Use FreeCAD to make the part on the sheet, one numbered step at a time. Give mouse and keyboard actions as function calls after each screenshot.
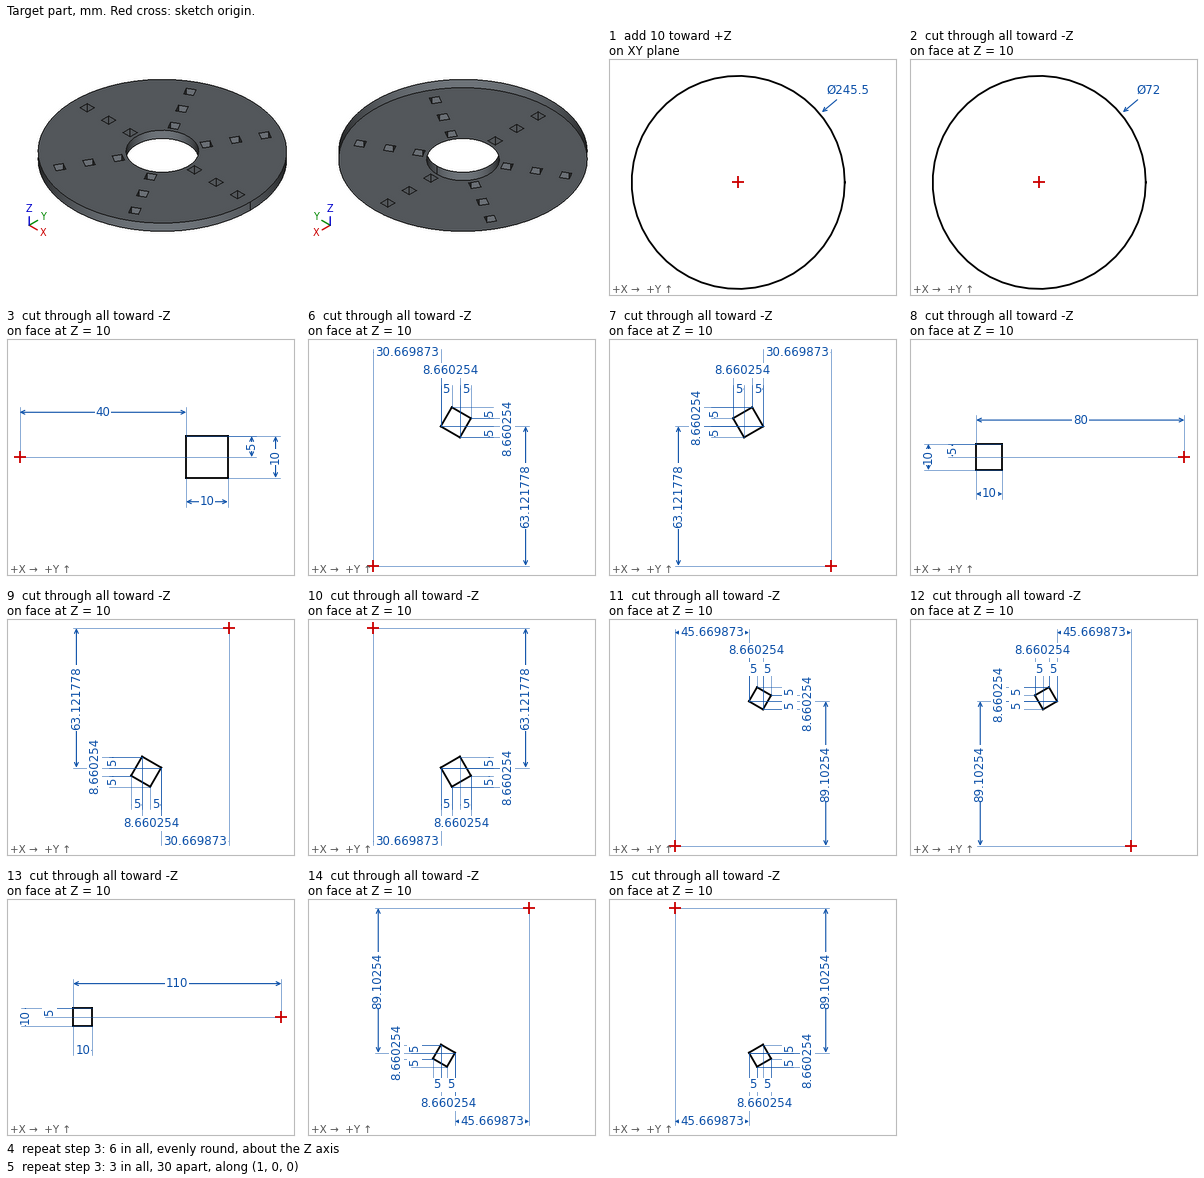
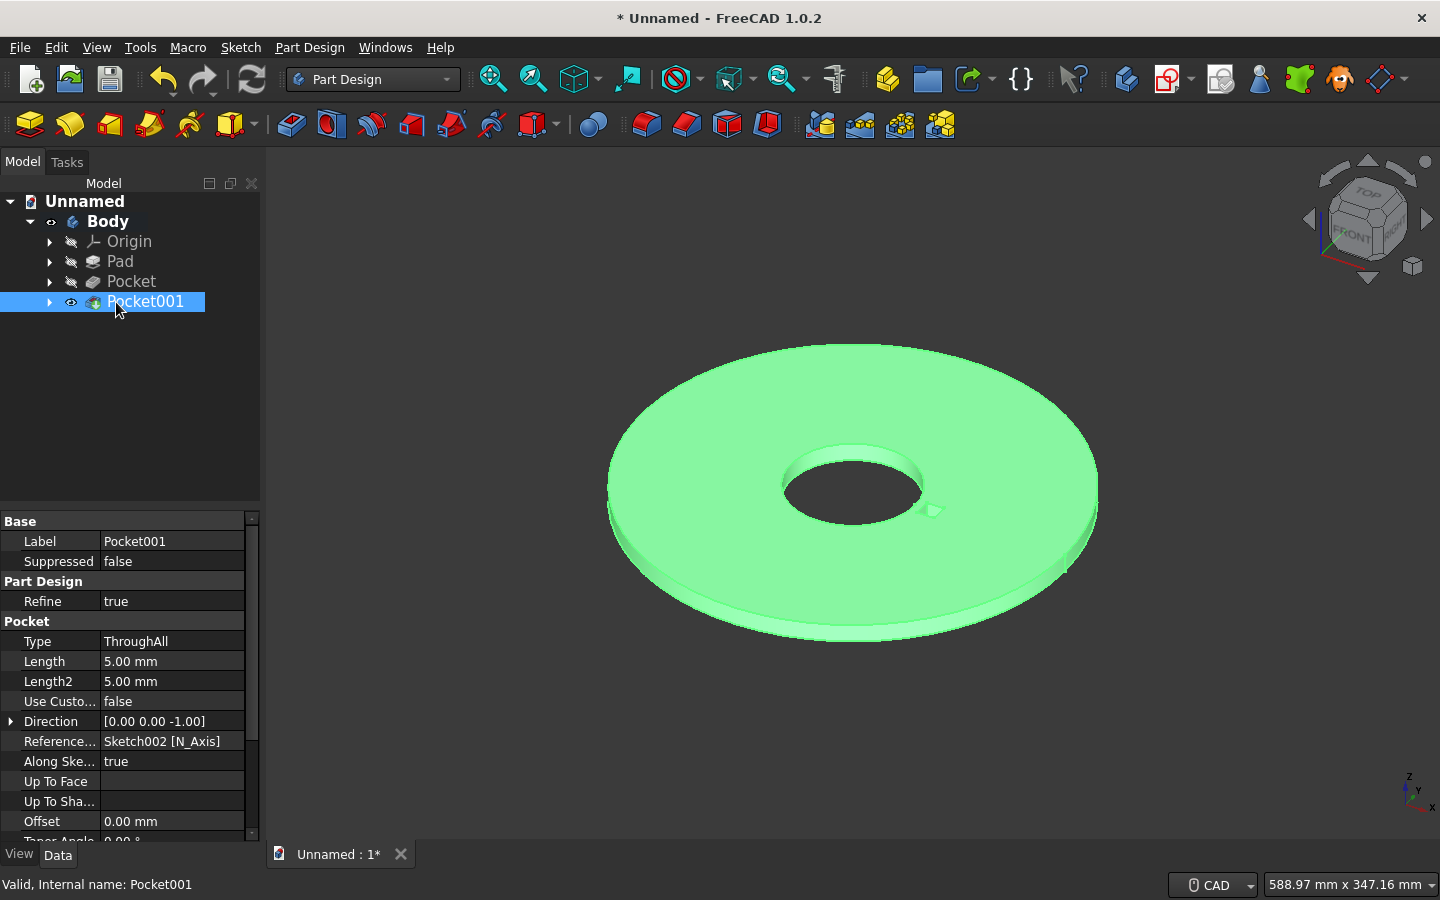
click(900, 124)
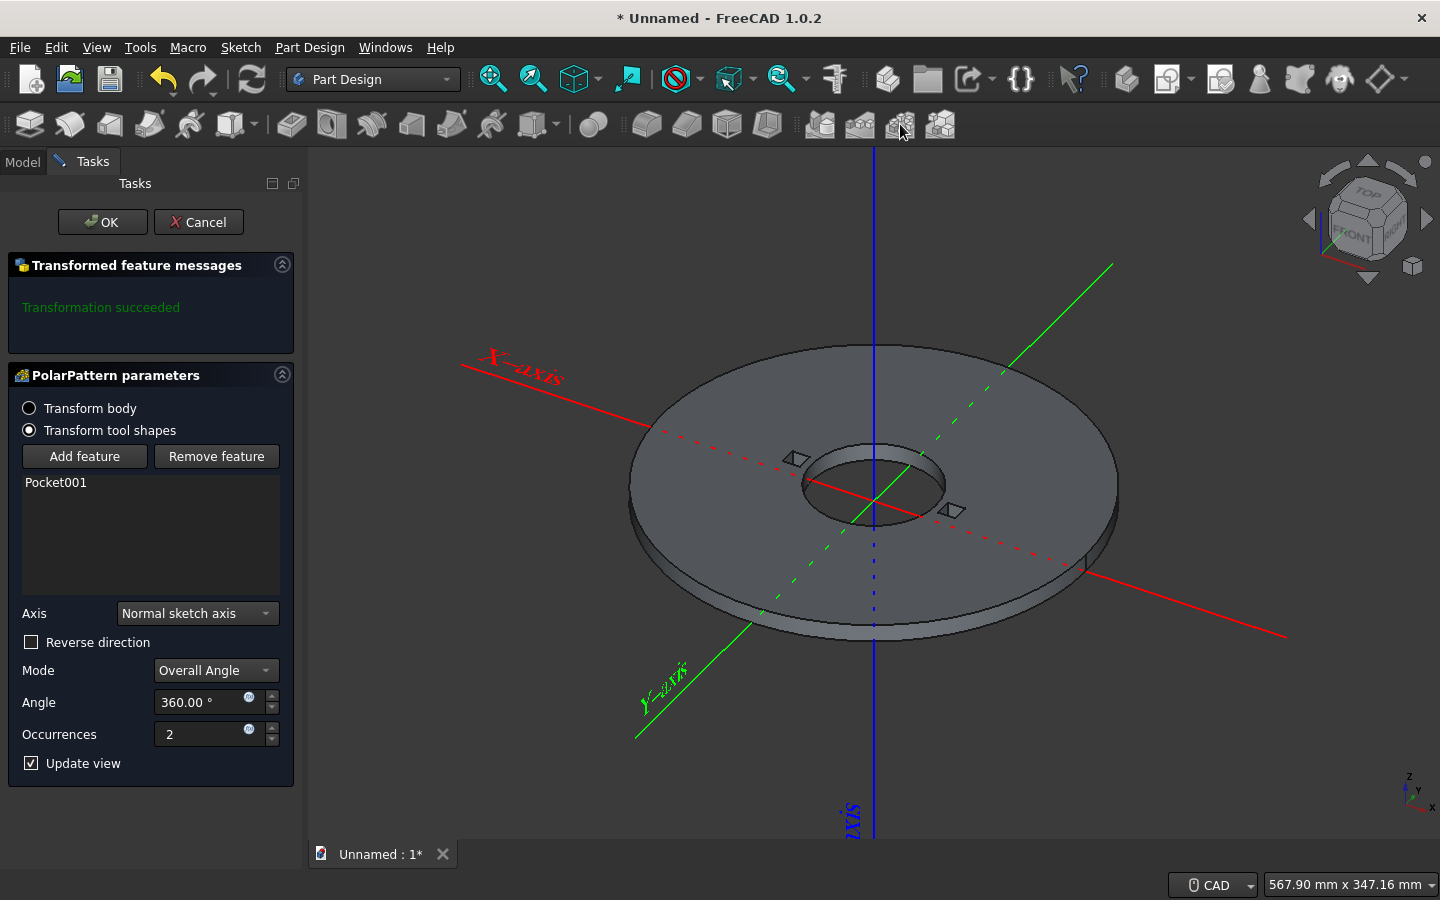
click(198, 614)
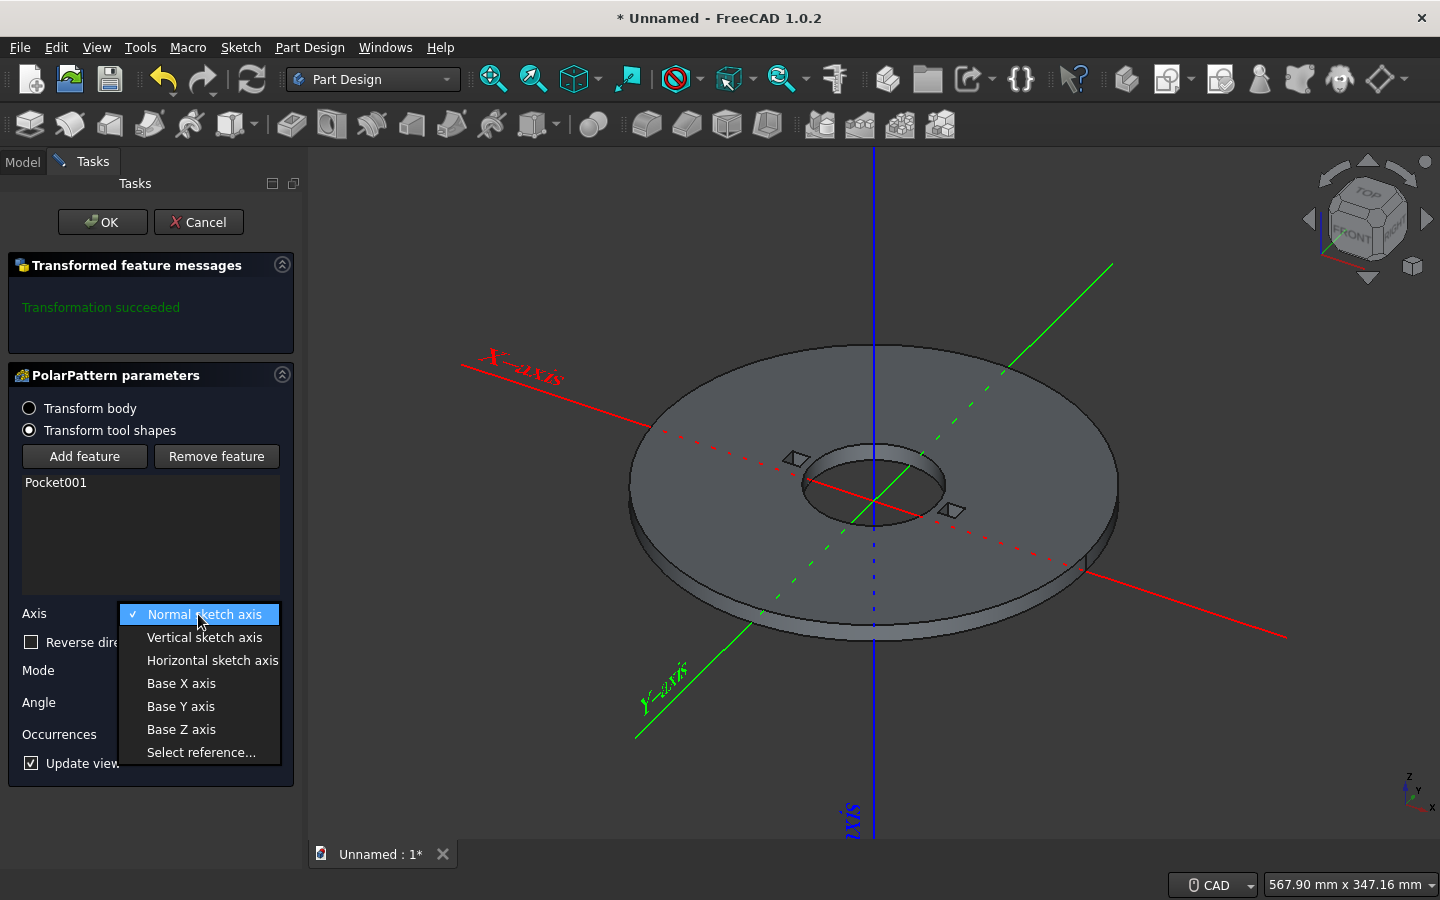
click(198, 730)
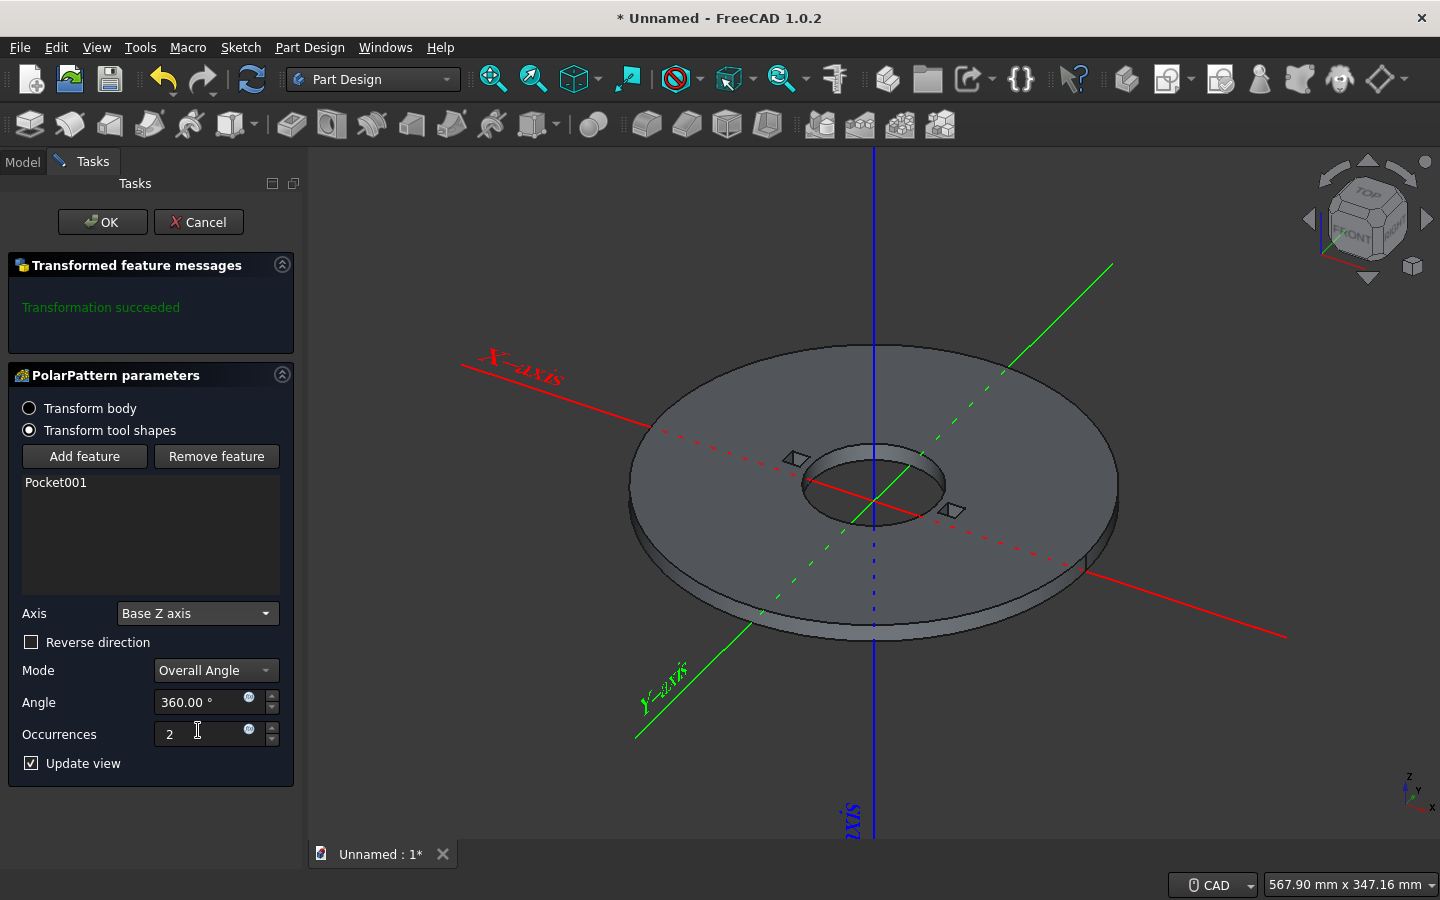
triple_click(209, 734)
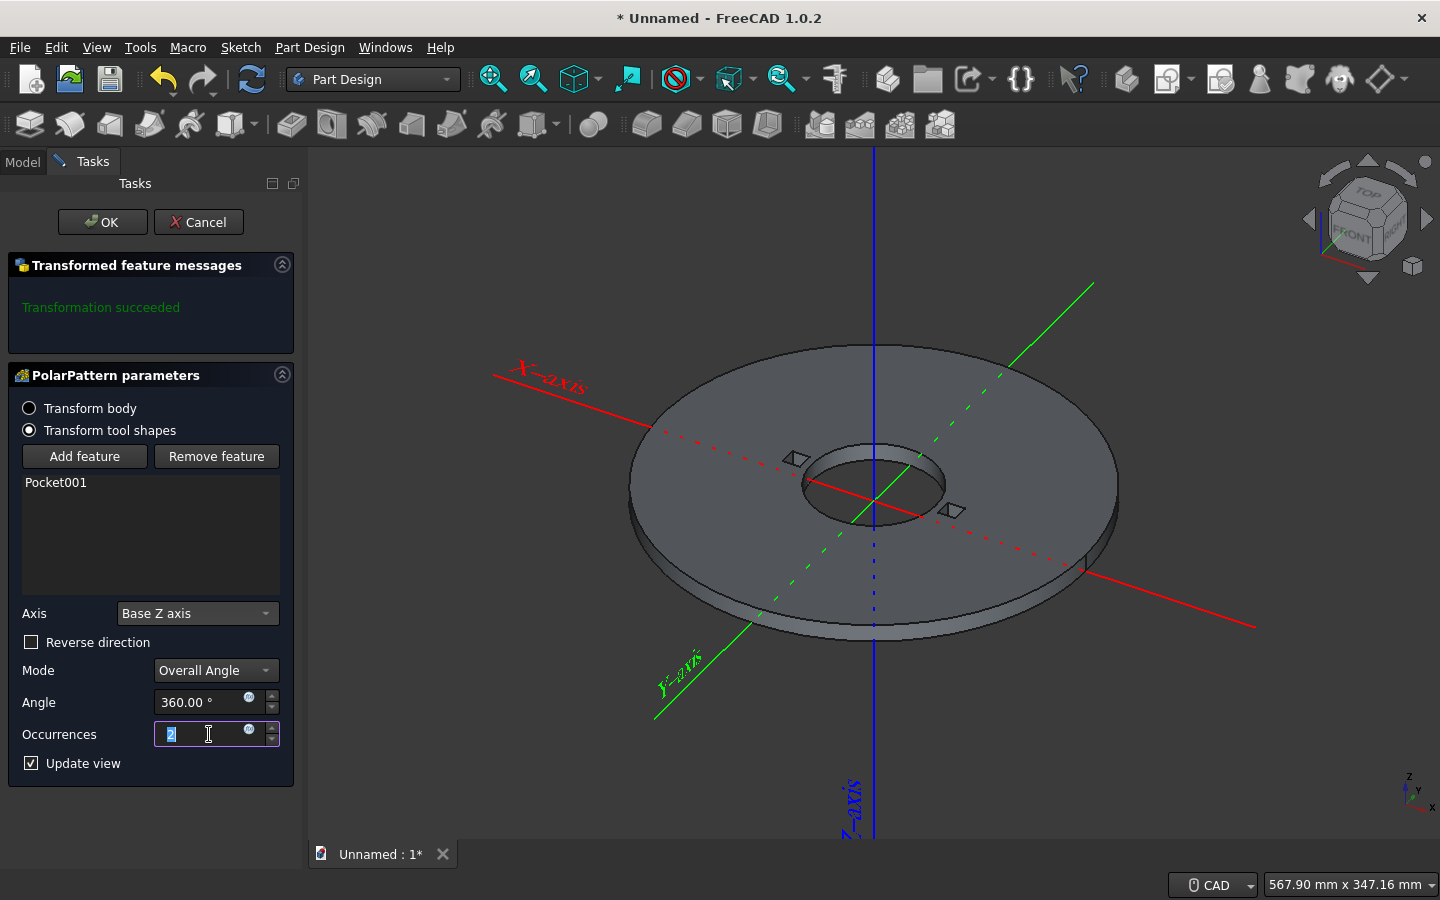
text(6)
key(Tab)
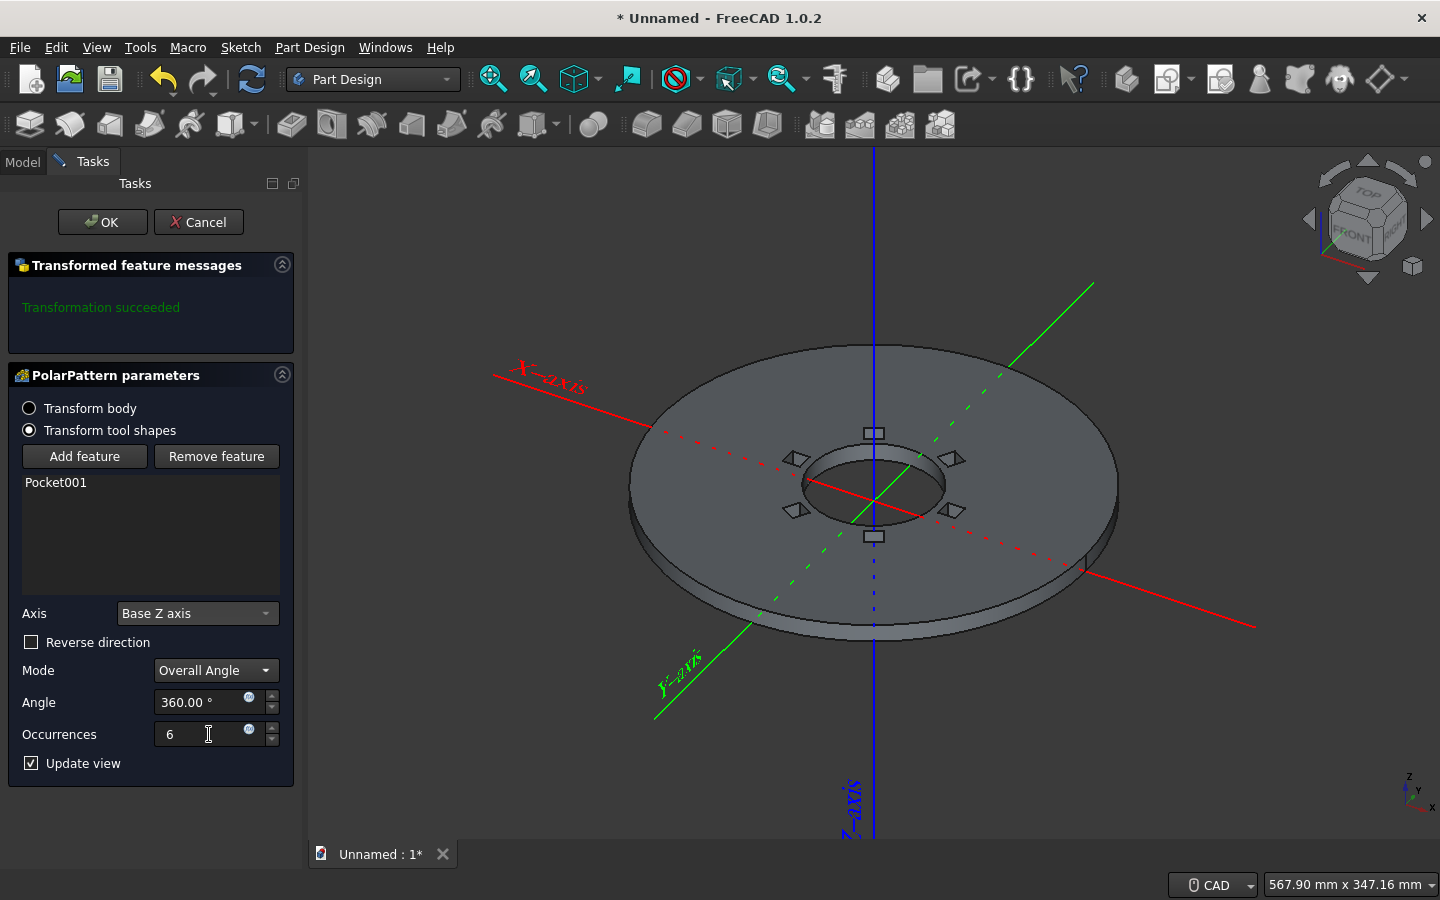
click(103, 222)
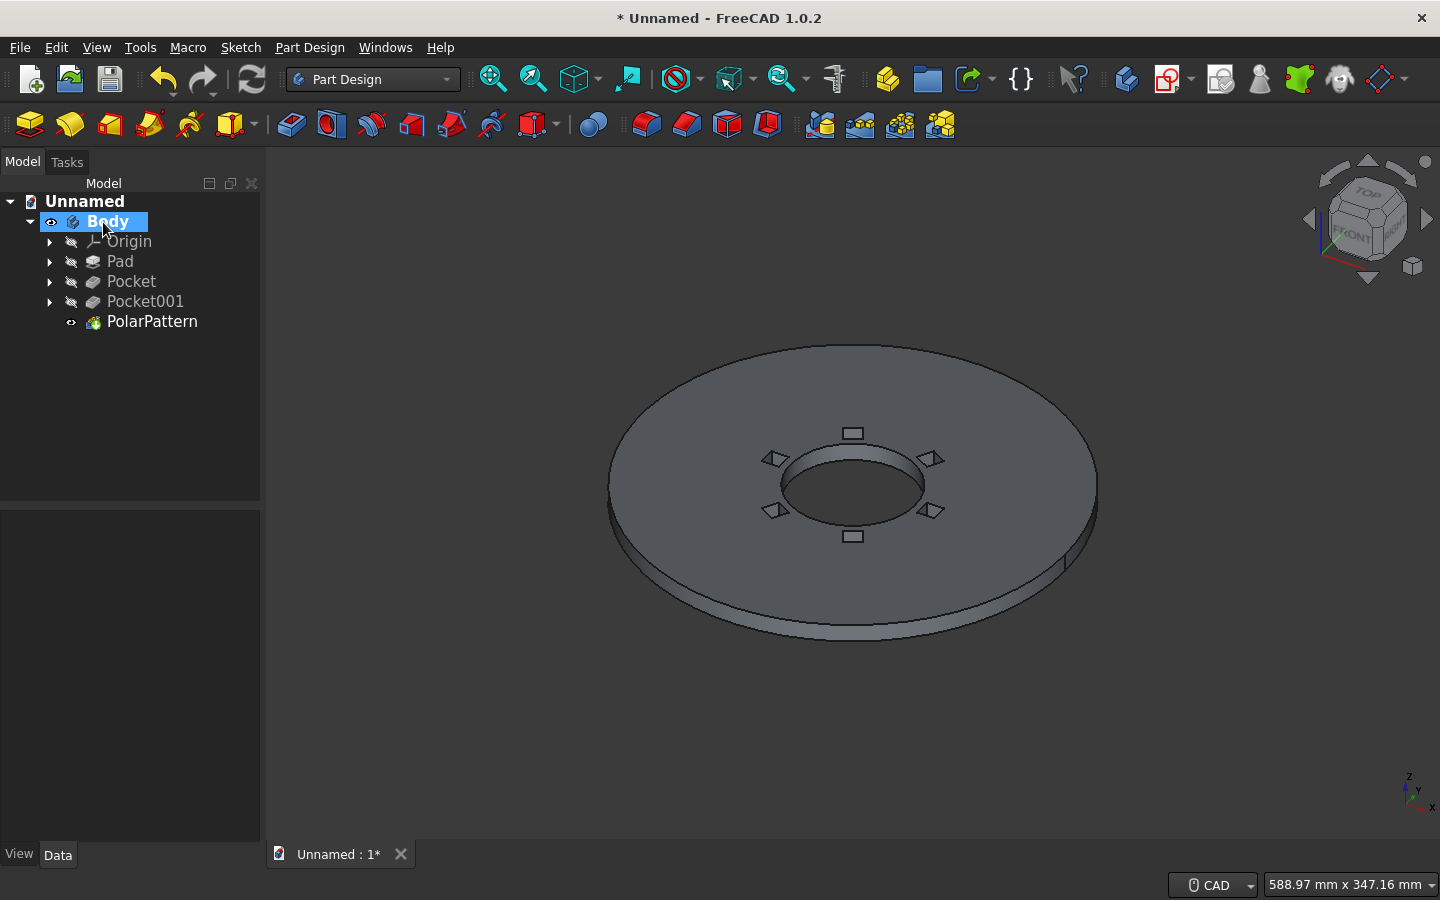
click(116, 302)